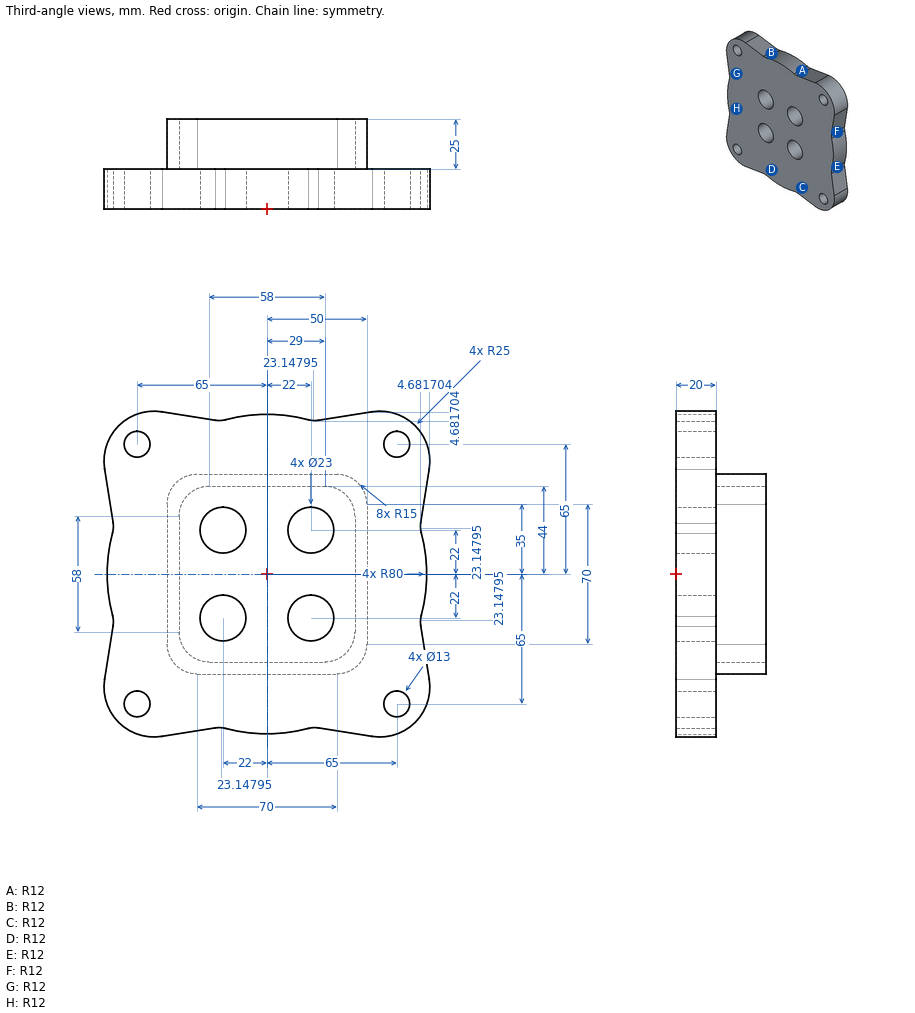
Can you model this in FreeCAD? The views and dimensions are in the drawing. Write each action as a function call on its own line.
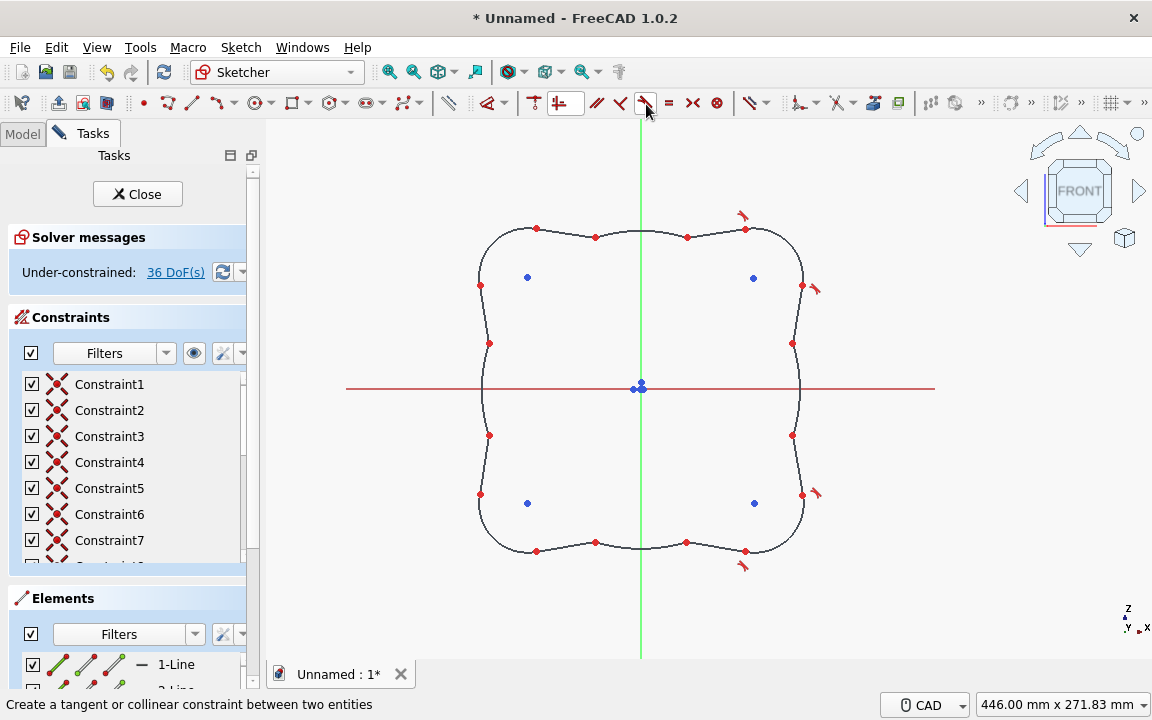
click(577, 545)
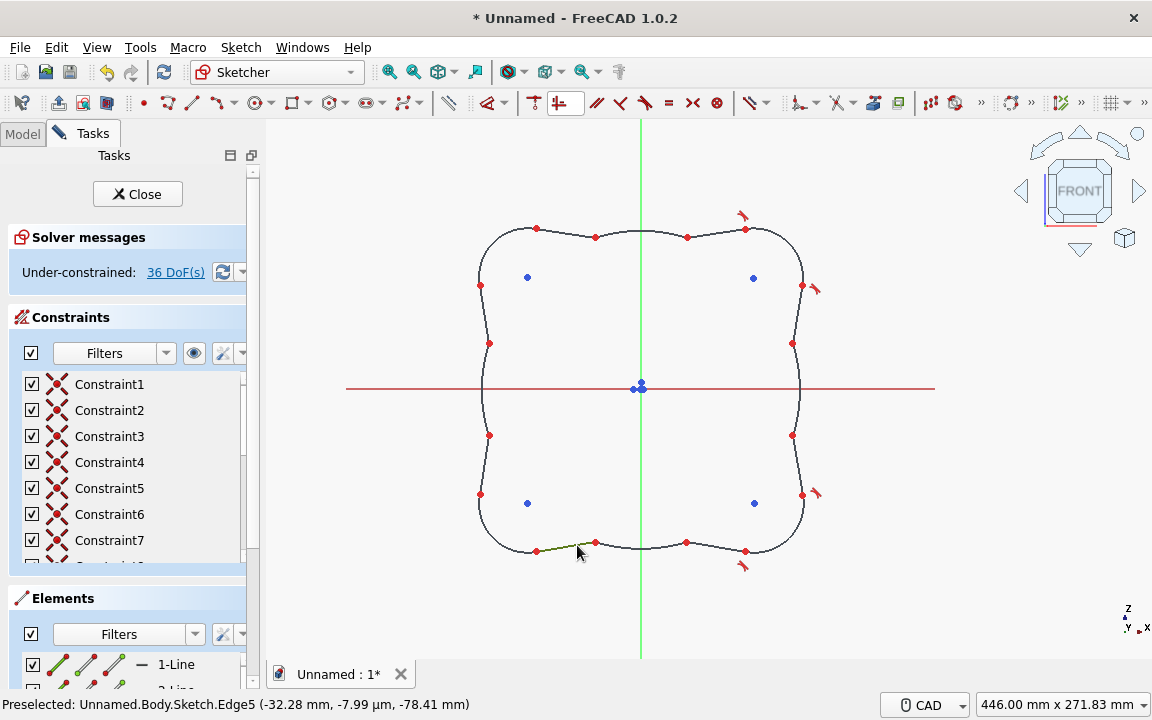
click(483, 523)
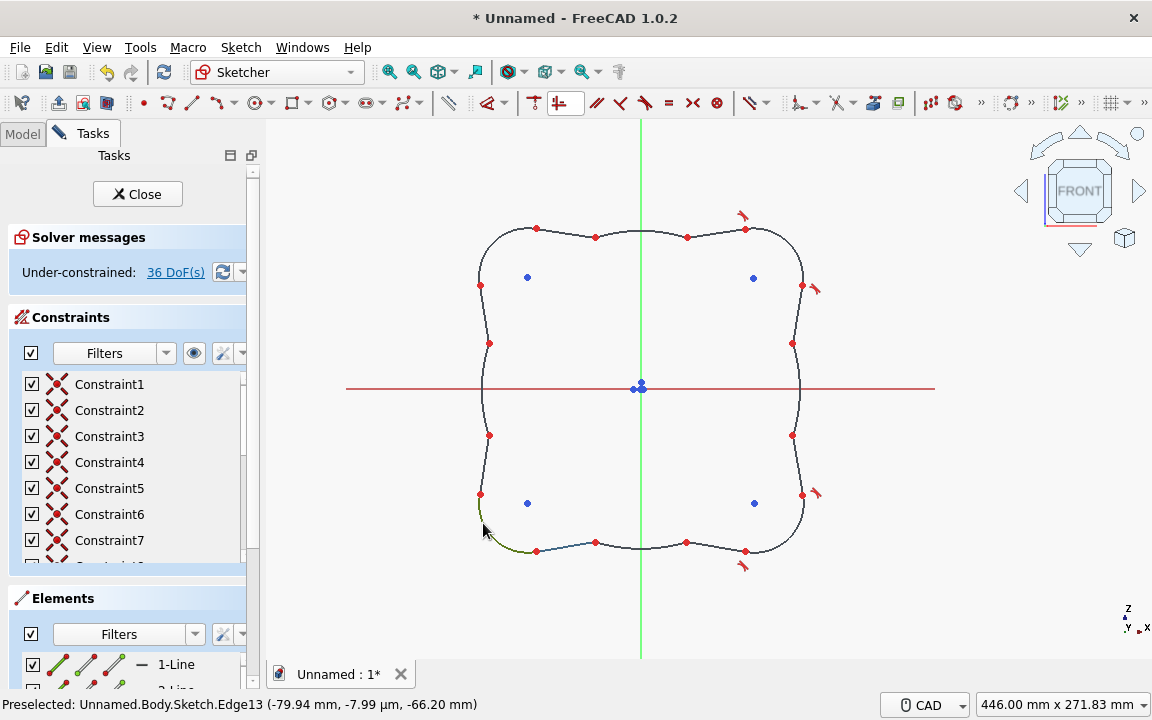
click(646, 104)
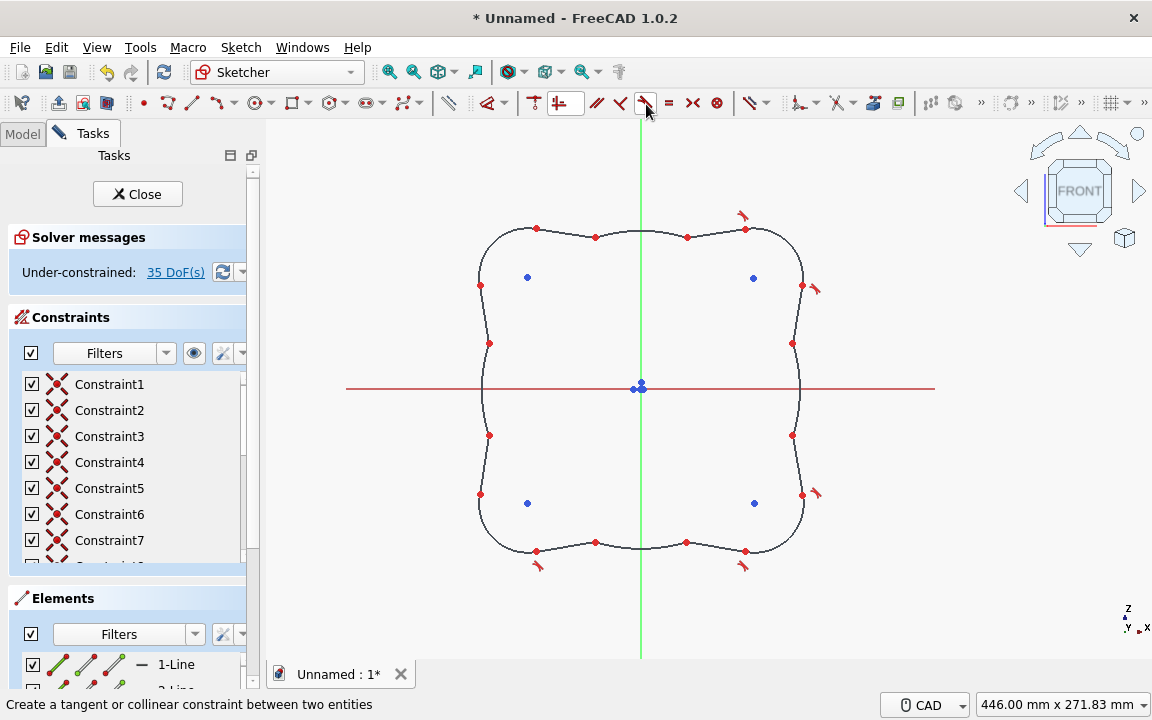
click(483, 477)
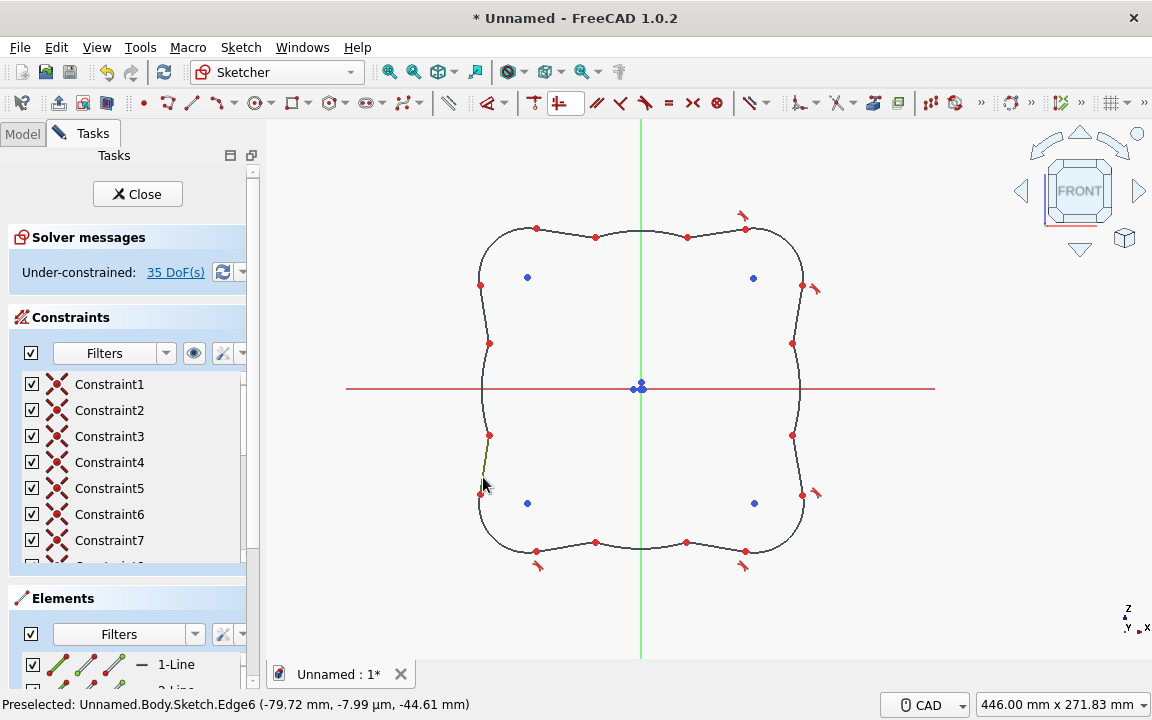
click(483, 523)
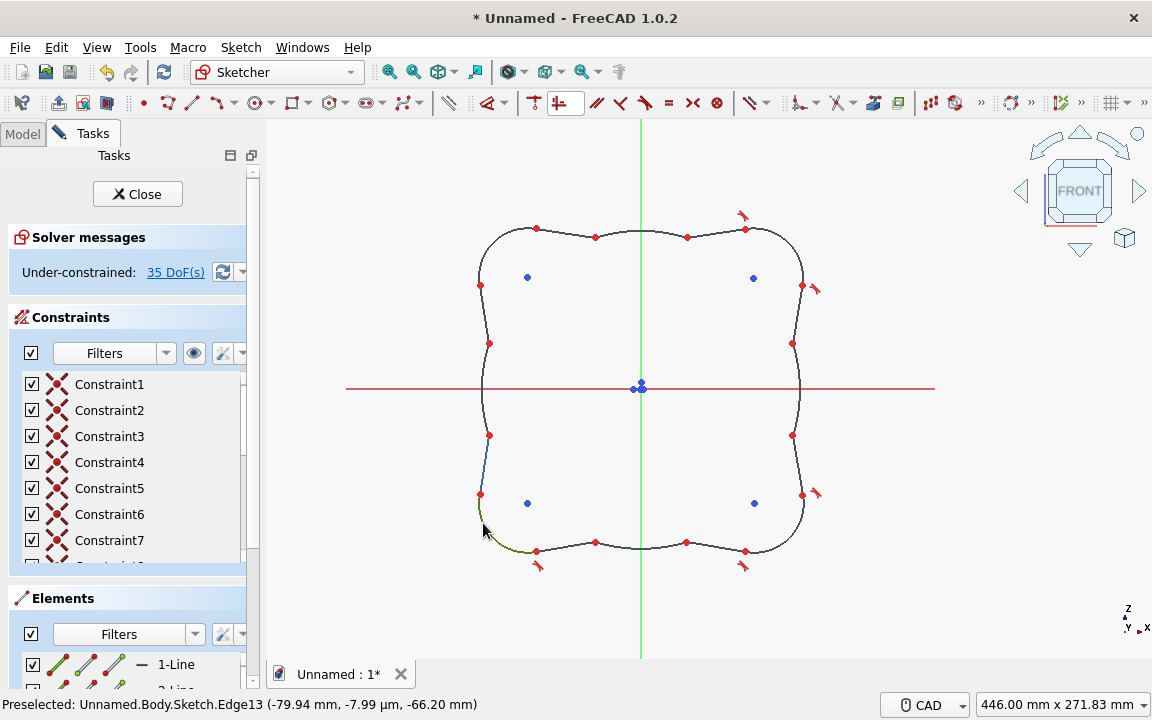
click(646, 104)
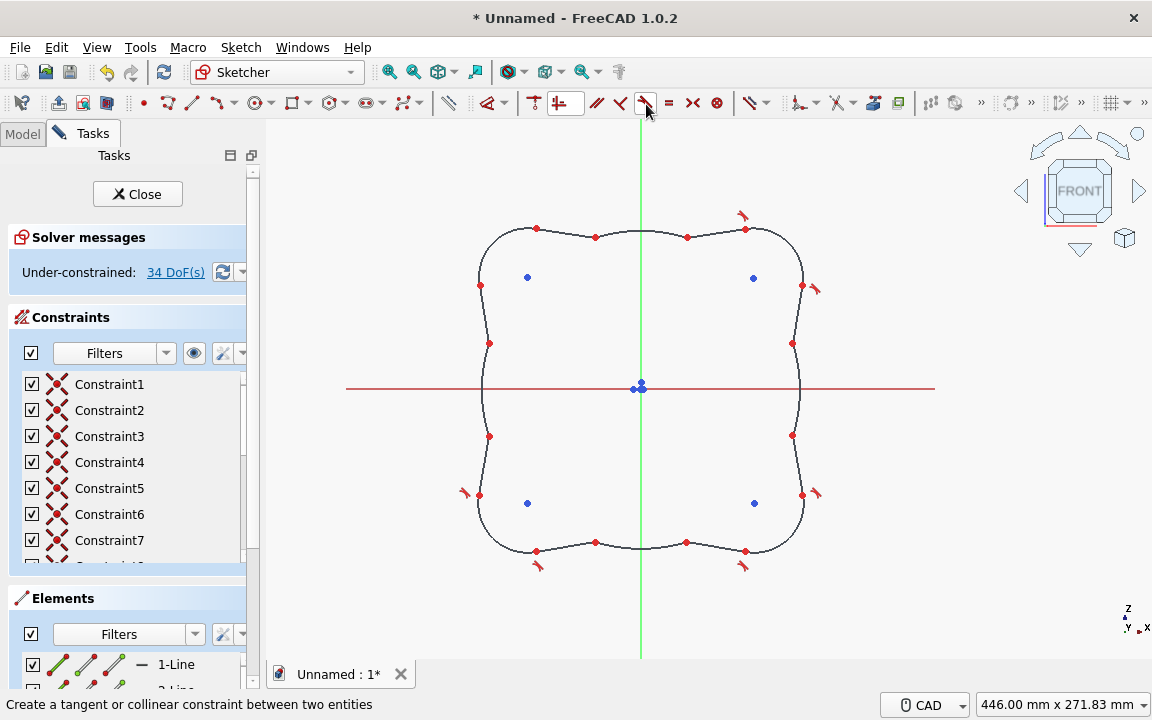
click(486, 327)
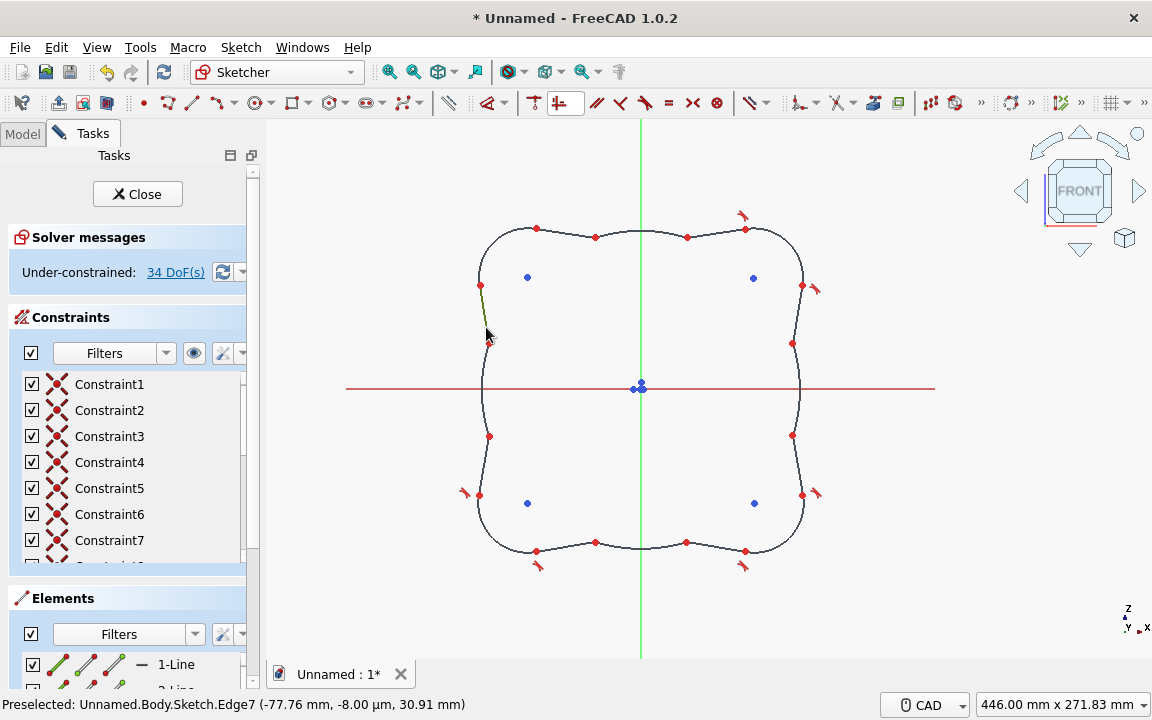
click(508, 232)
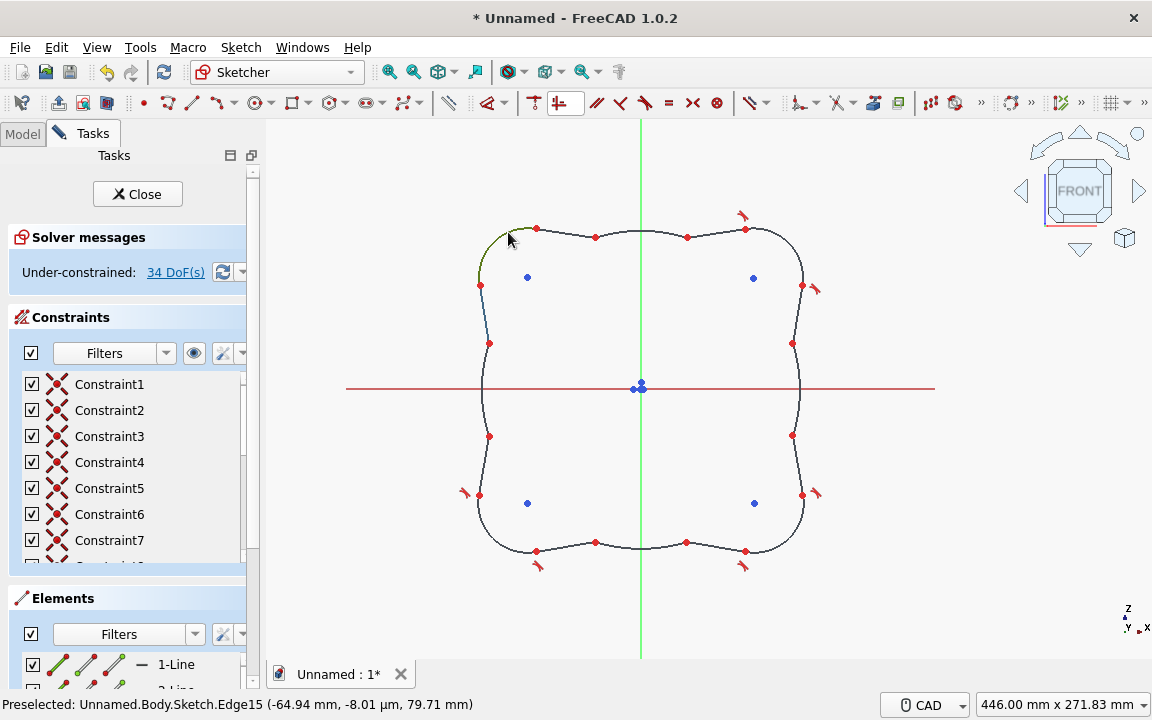
click(646, 104)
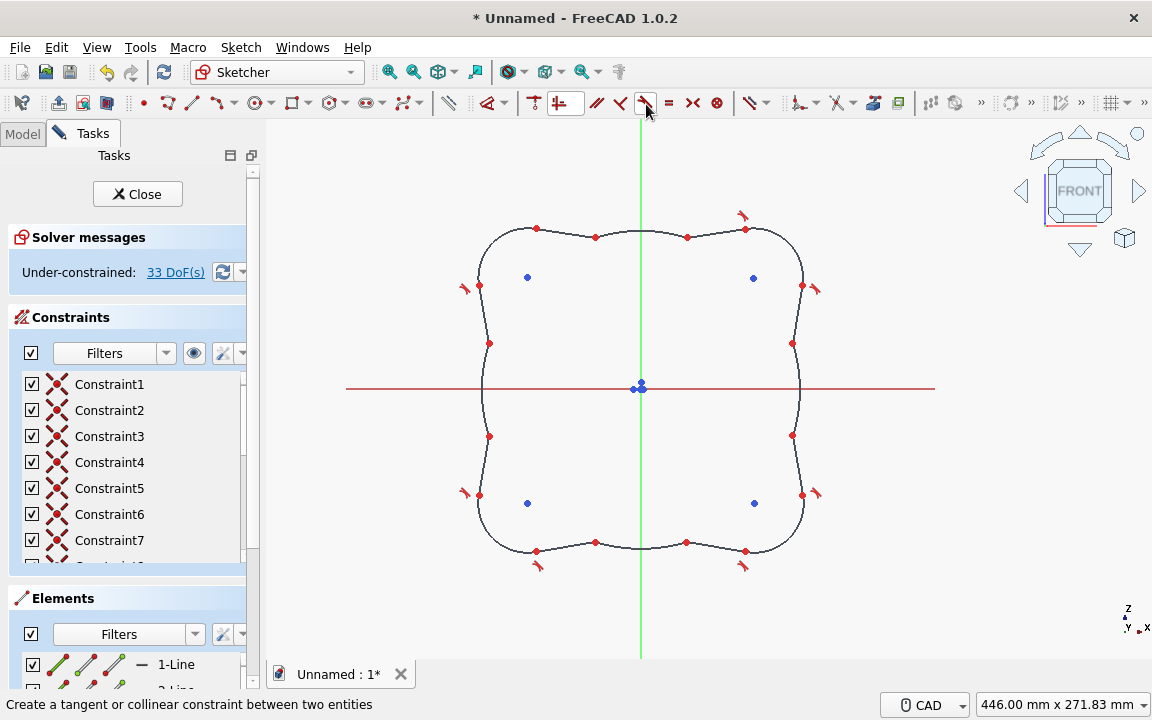
click(554, 232)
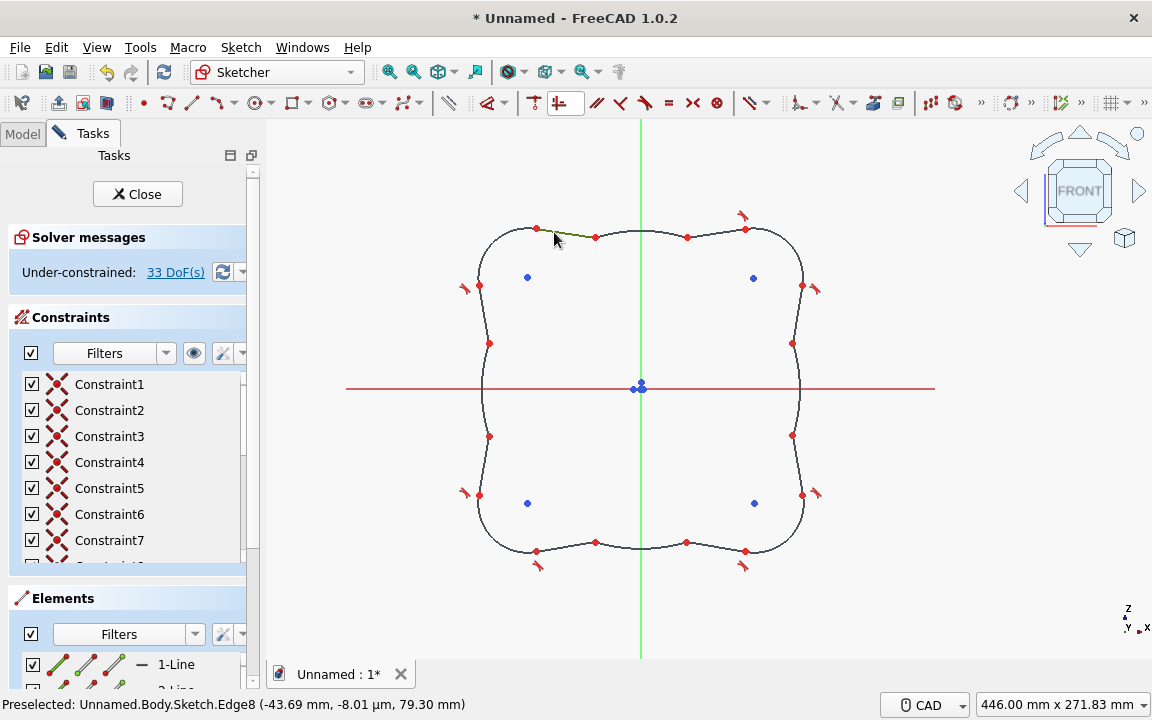
click(508, 232)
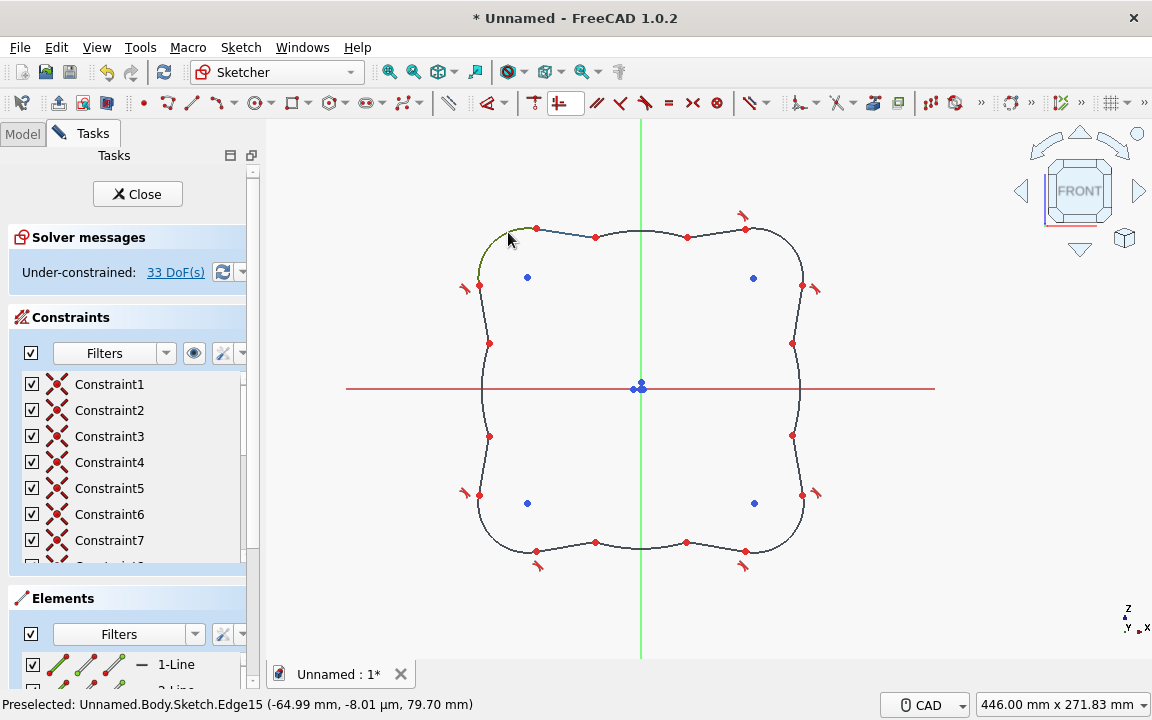
click(646, 104)